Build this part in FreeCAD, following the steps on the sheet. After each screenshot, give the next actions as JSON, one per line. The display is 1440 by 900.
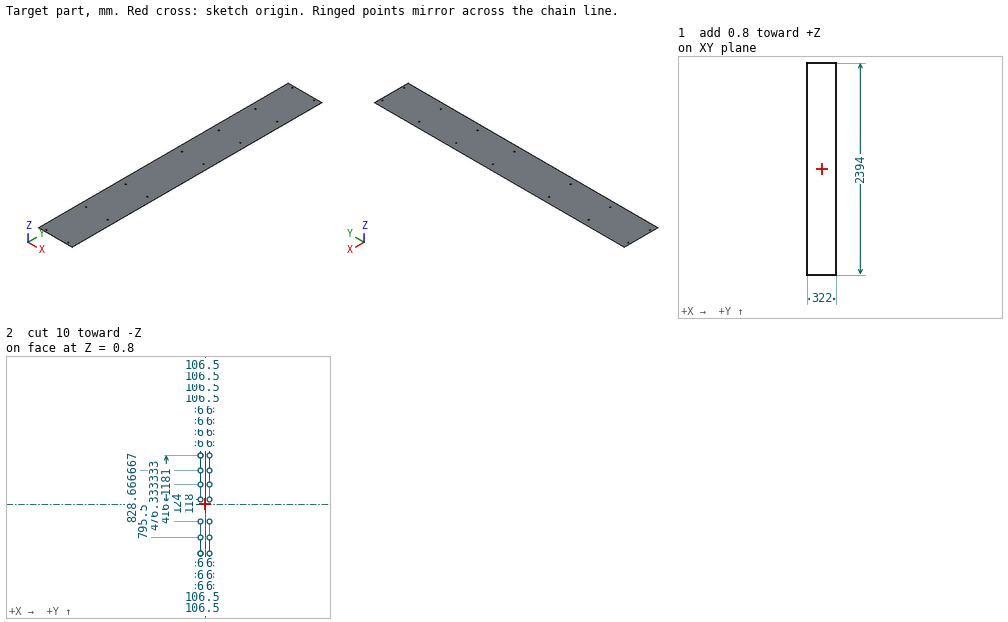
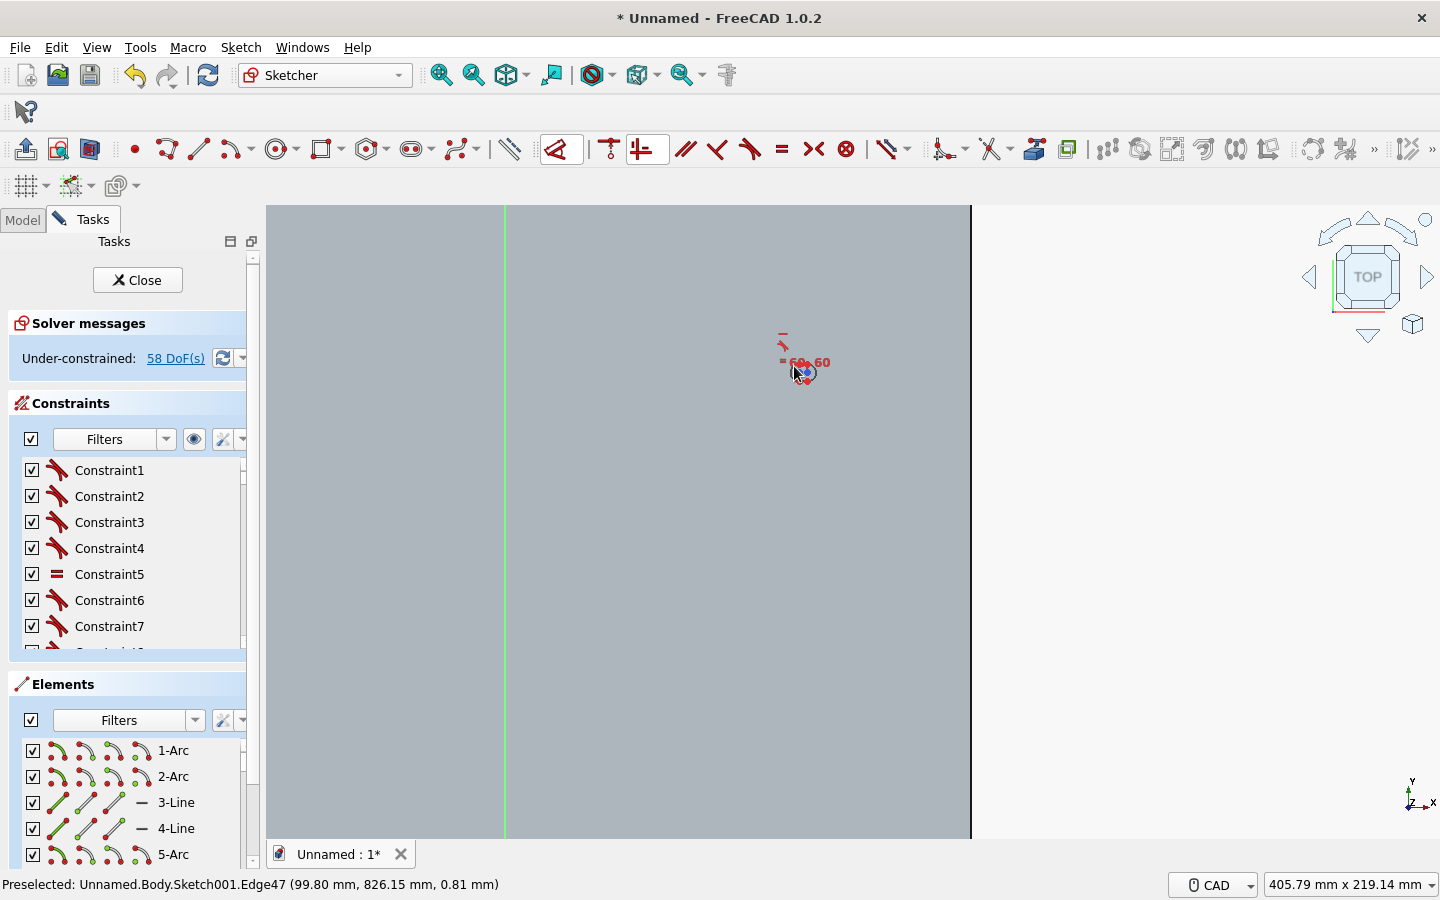
{"action": "scroll", "coordinate": [803, 377], "scroll_direction": "down", "scroll_amount": 14}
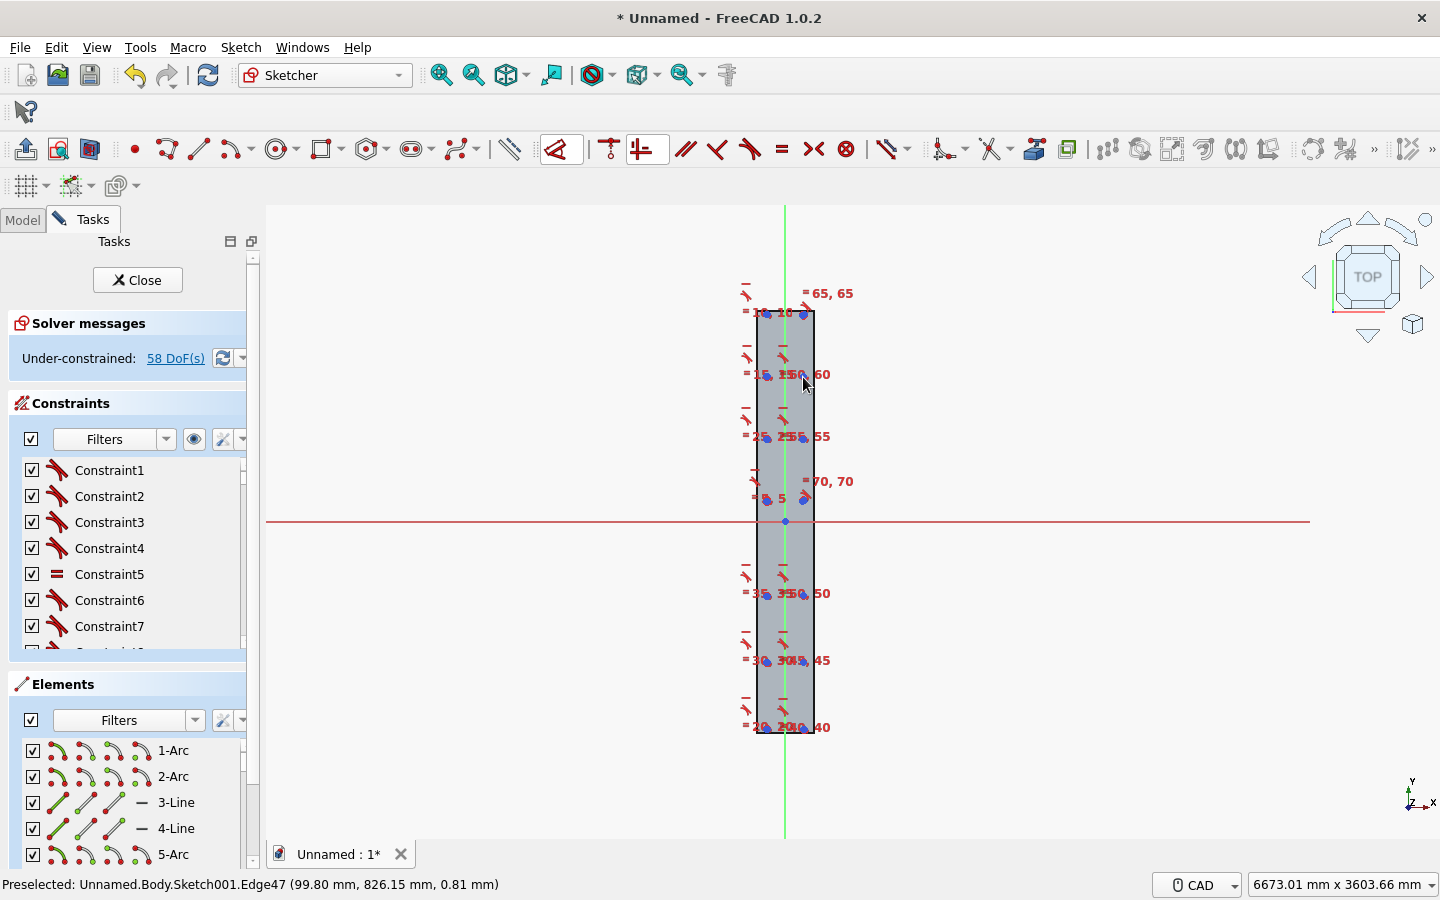
{"action": "scroll", "coordinate": [803, 315], "scroll_direction": "up", "scroll_amount": 14}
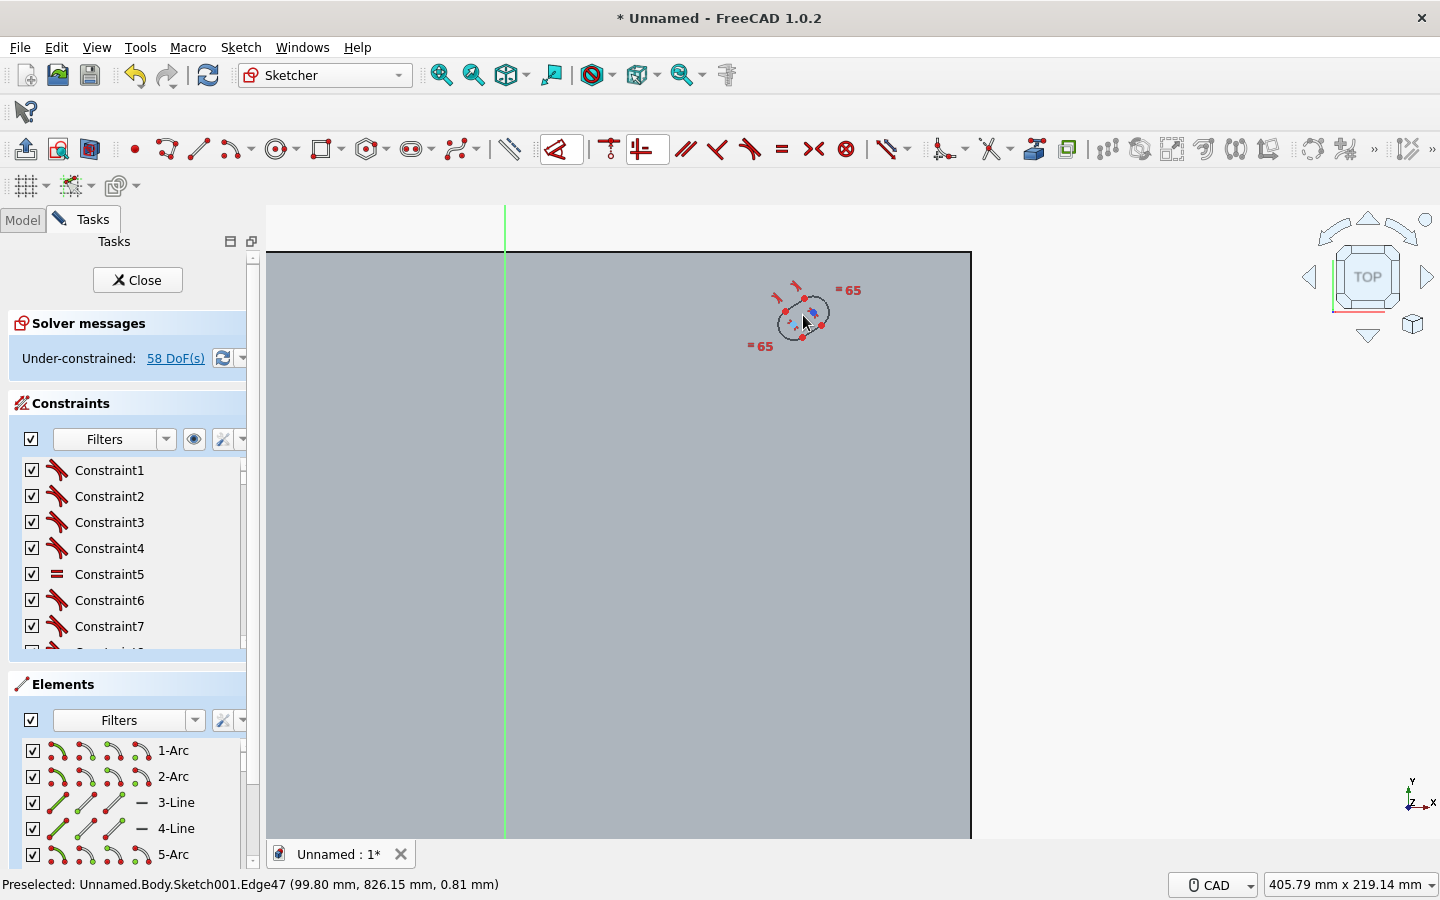
{"action": "left_click", "coordinate": [793, 306]}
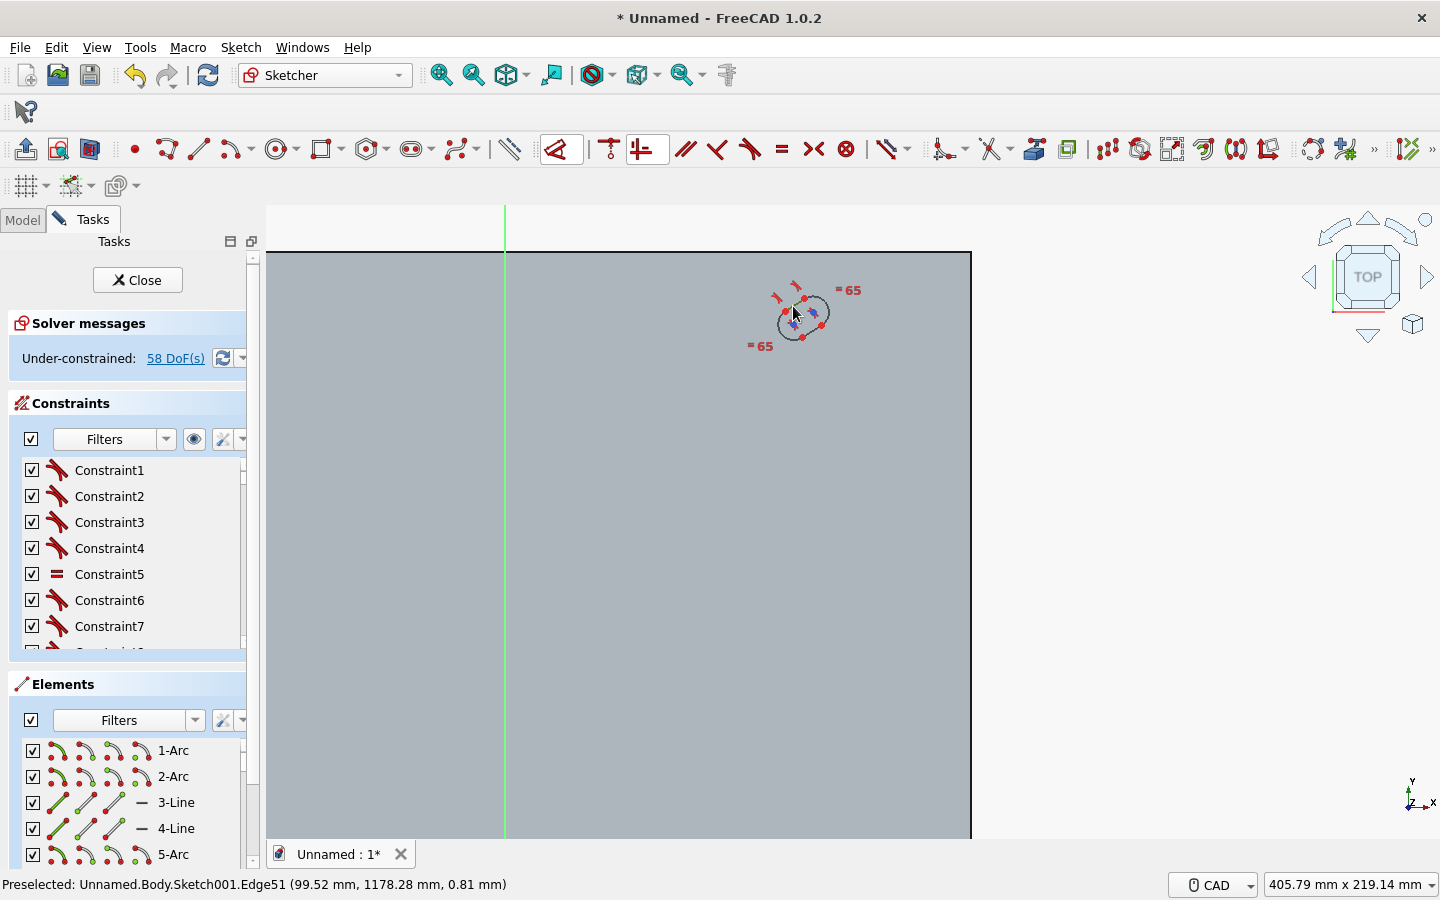
{"action": "key", "text": "h"}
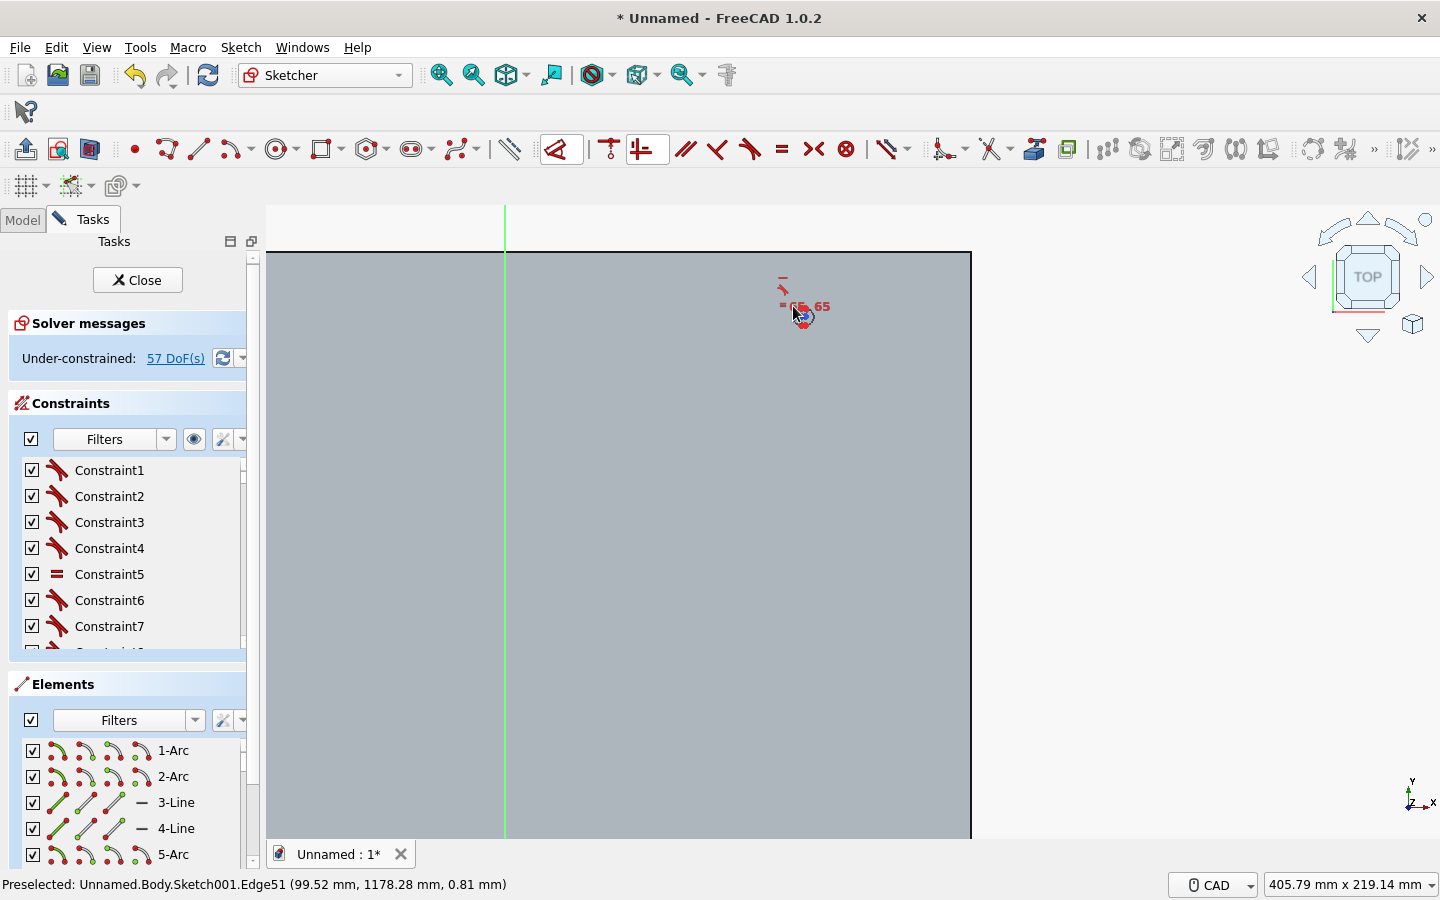
{"action": "scroll", "coordinate": [803, 315], "scroll_direction": "down", "scroll_amount": 14}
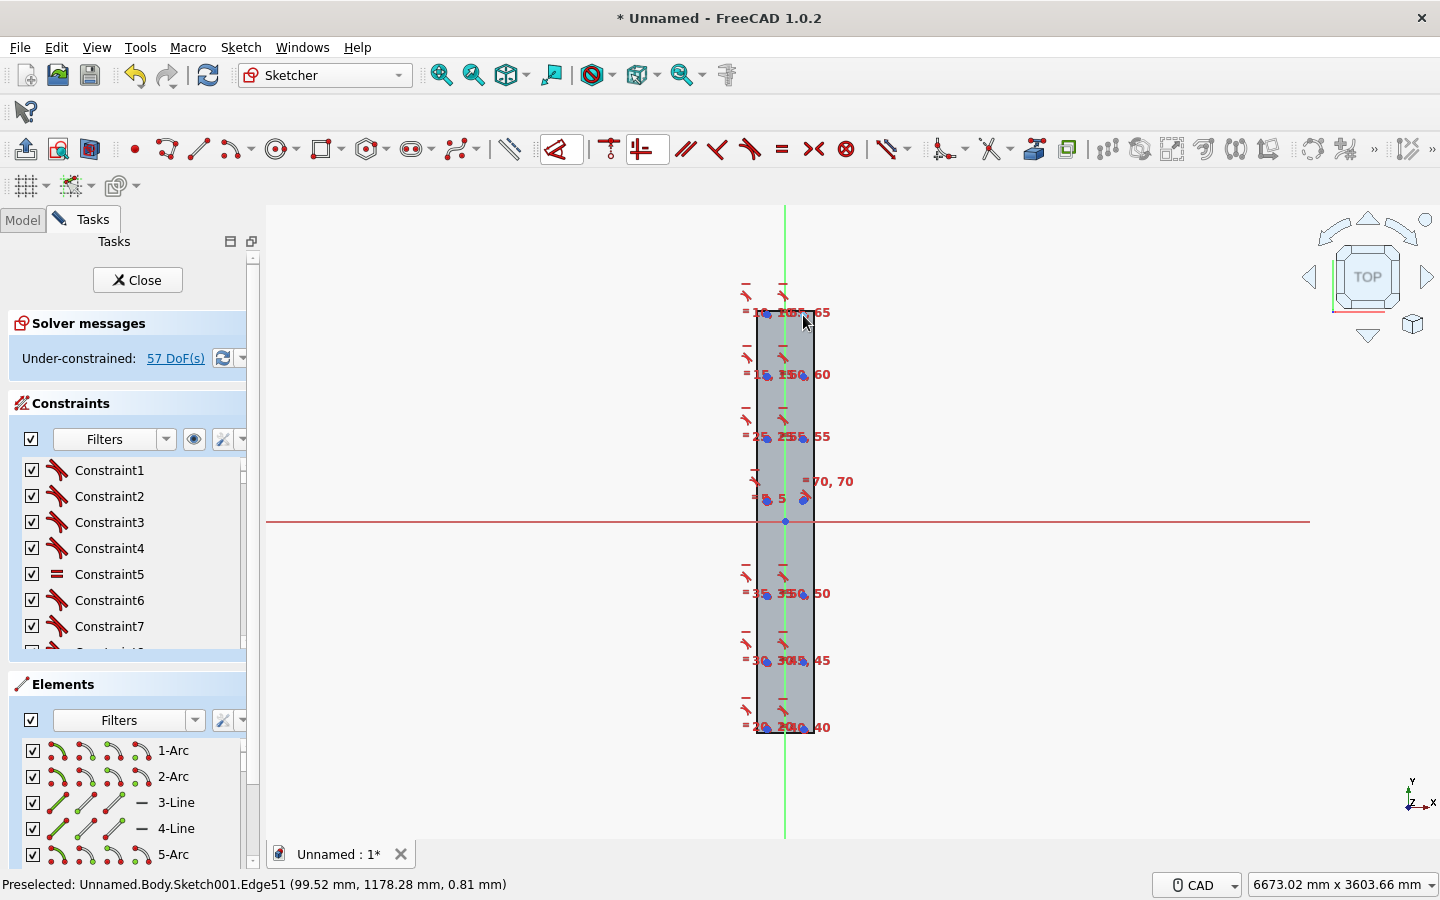
{"action": "scroll", "coordinate": [803, 500], "scroll_direction": "up", "scroll_amount": 14}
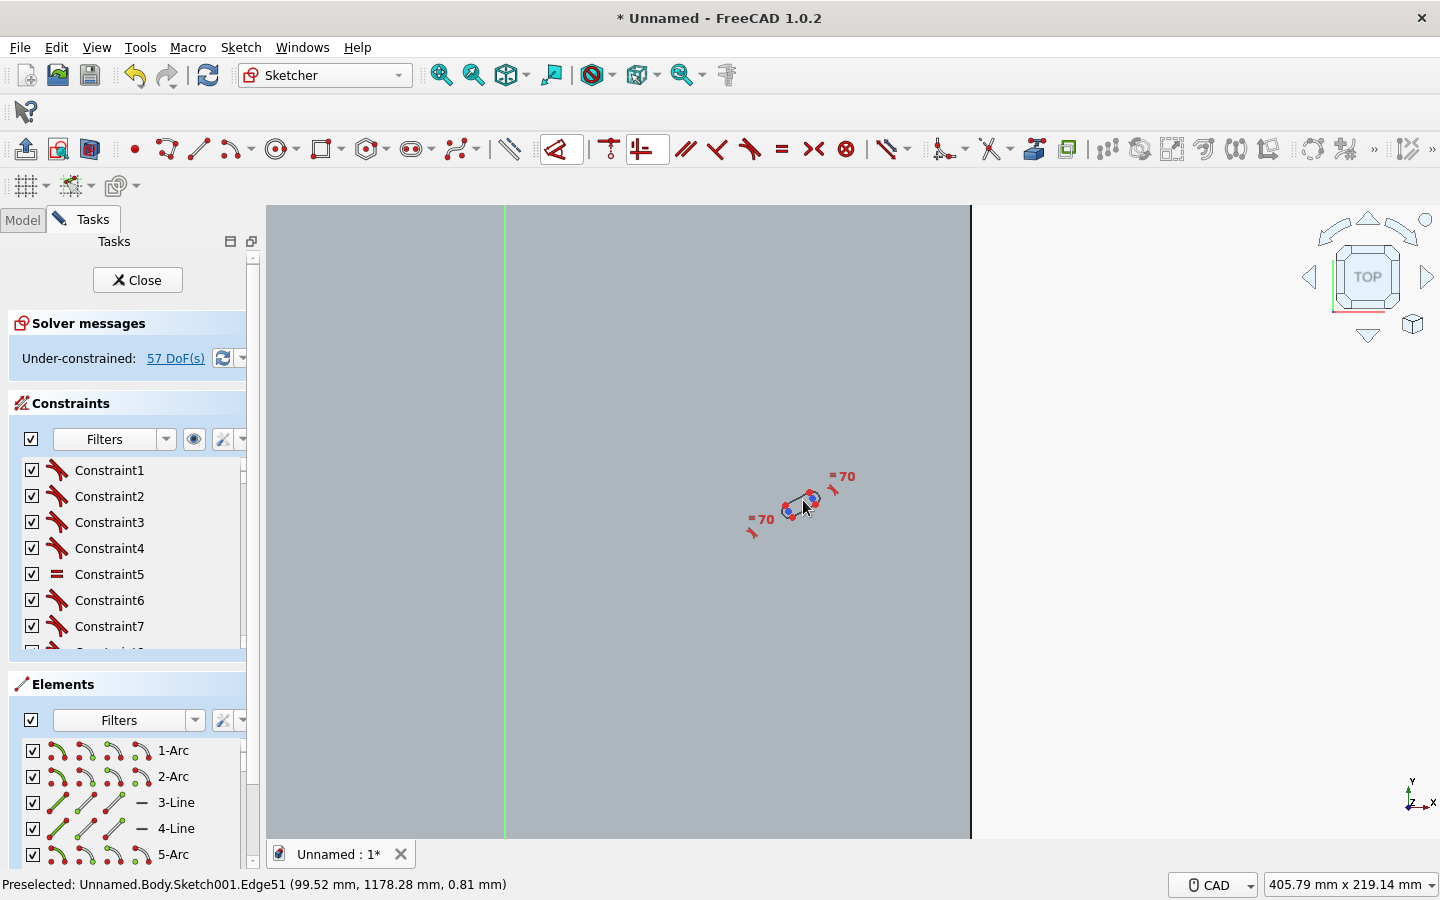
{"action": "left_click", "coordinate": [795, 500]}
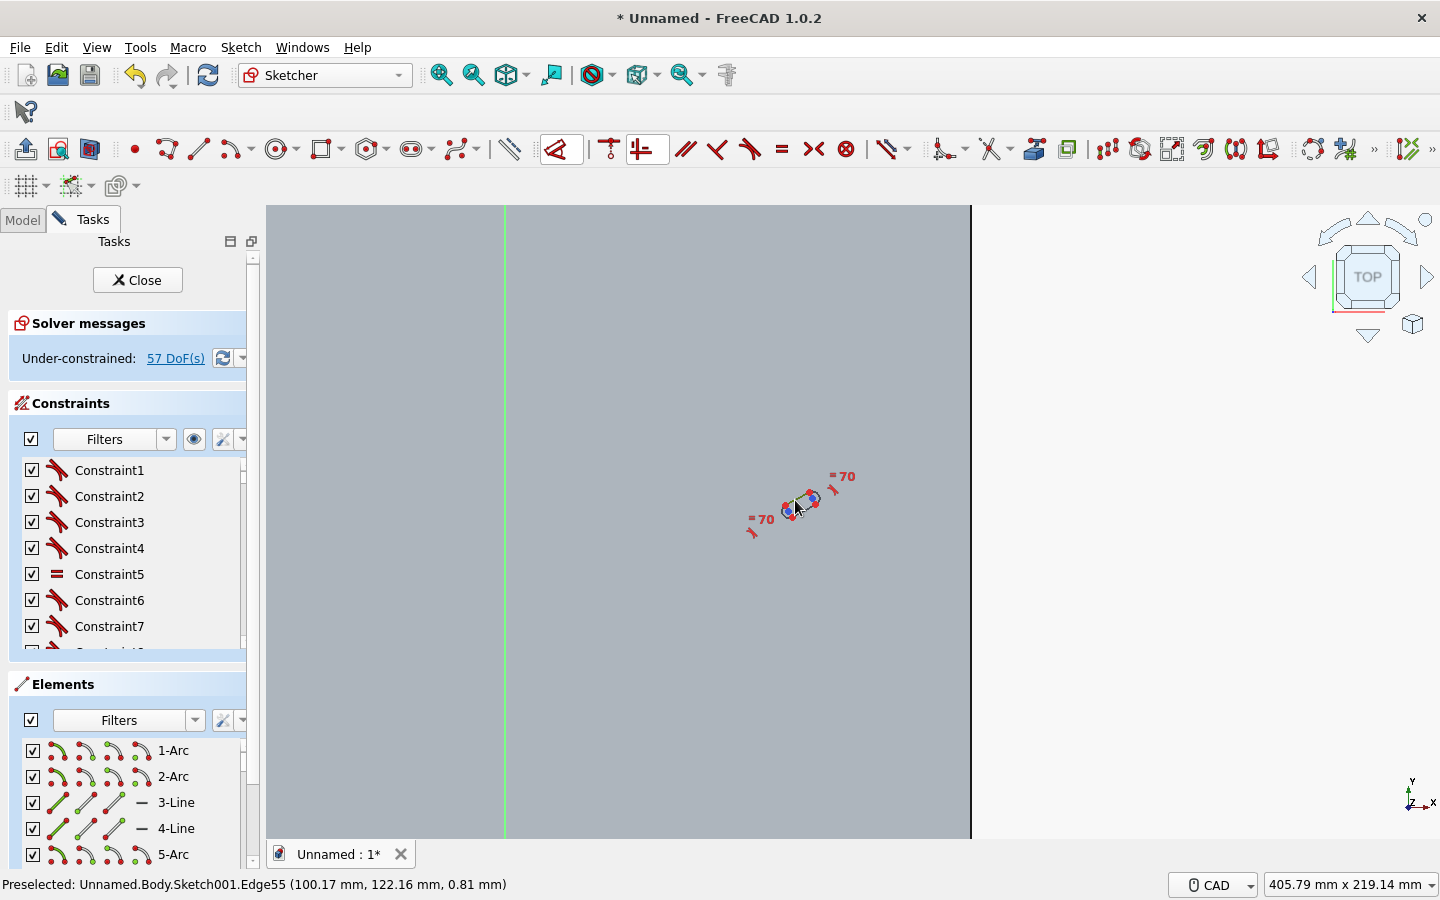
{"action": "key", "text": "h"}